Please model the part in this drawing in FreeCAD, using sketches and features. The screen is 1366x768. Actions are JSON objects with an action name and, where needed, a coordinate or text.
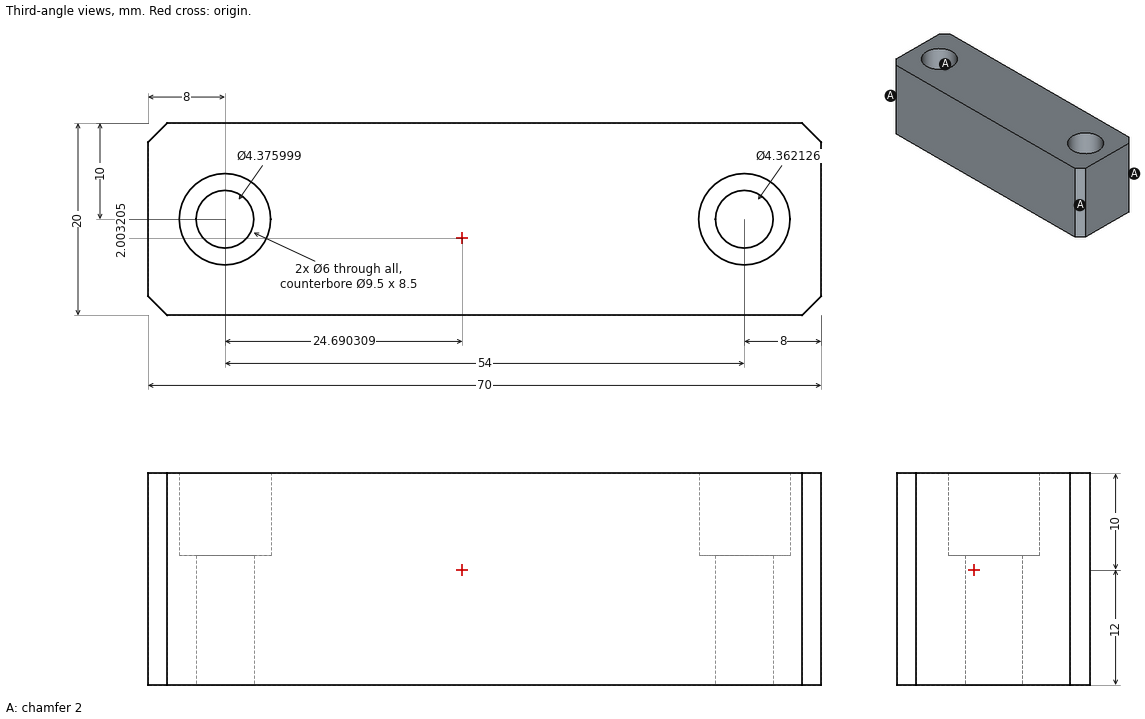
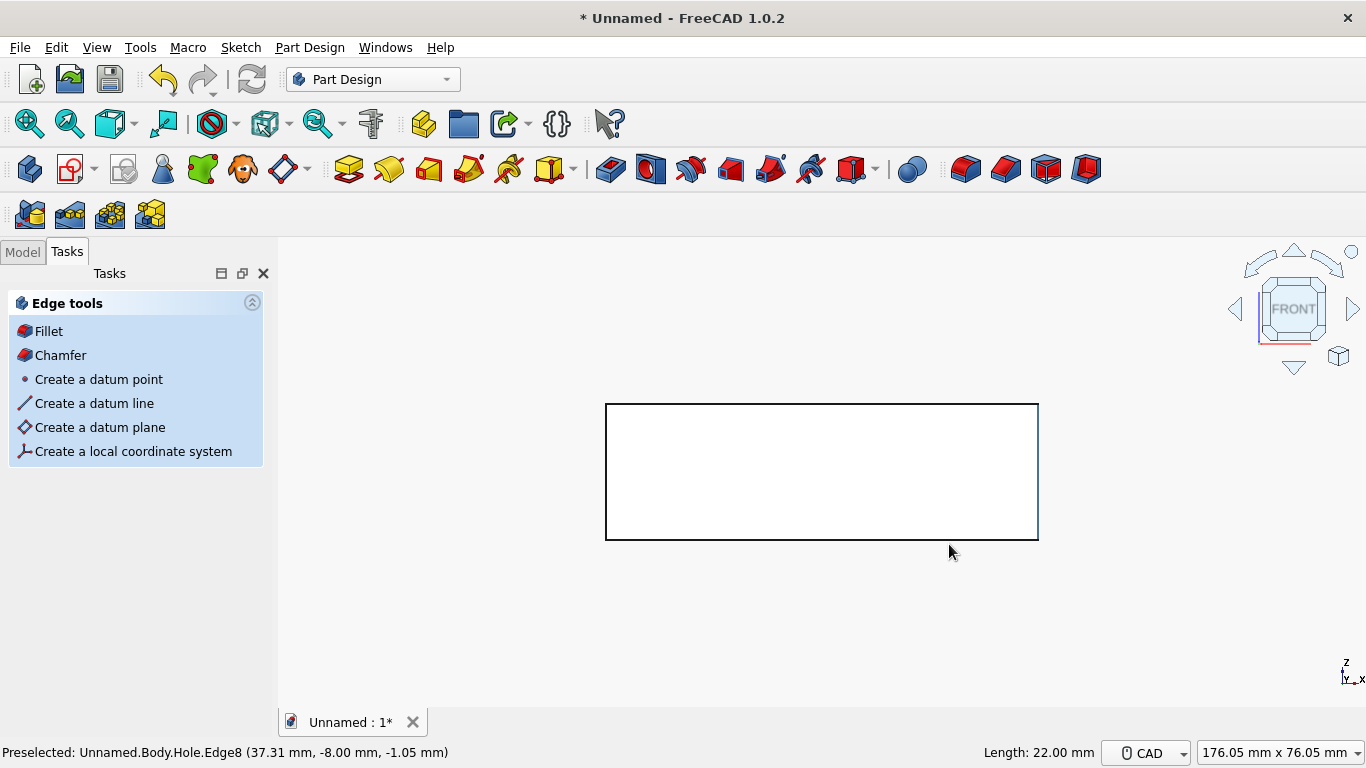
{"action": "left_click", "coordinate": [30, 124]}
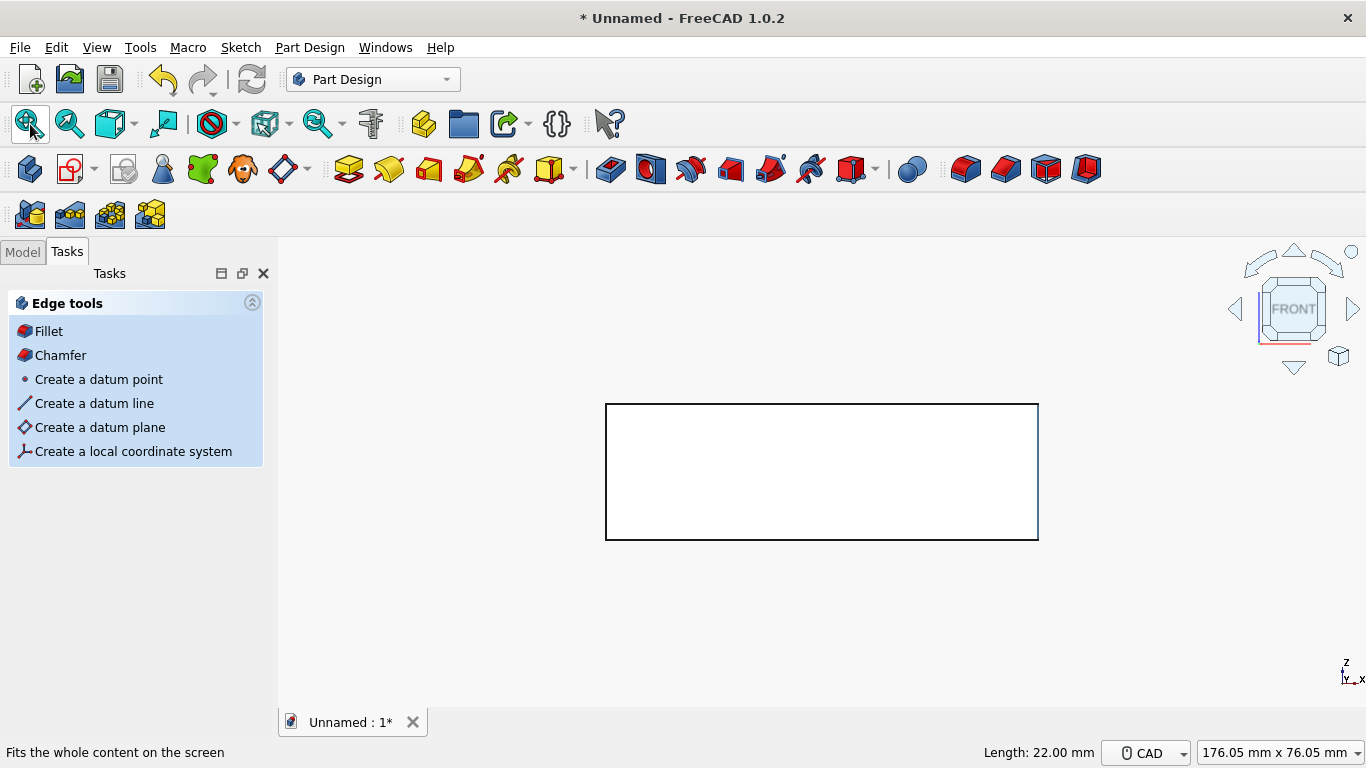
{"action": "left_click", "coordinate": [606, 471], "text": "ctrl"}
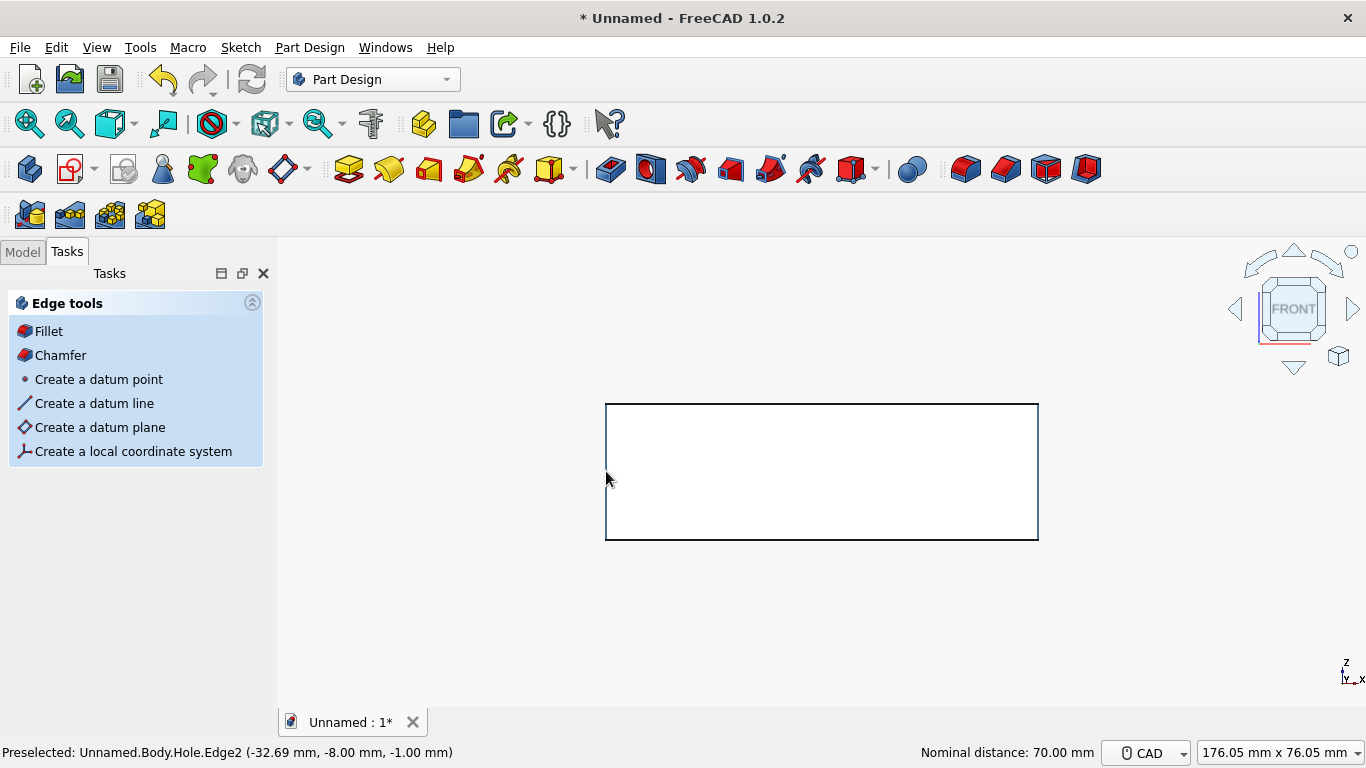
{"action": "key", "text": "3"}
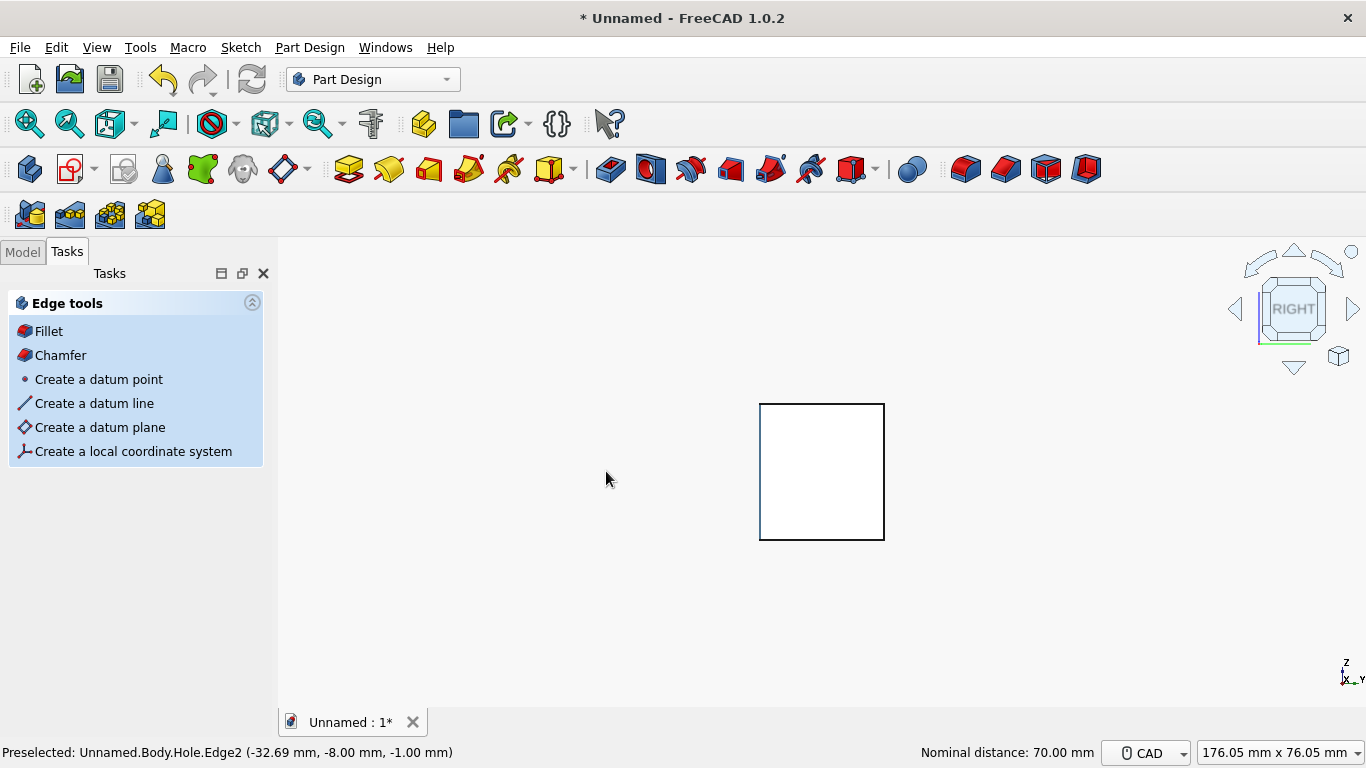
{"action": "key", "text": "v f"}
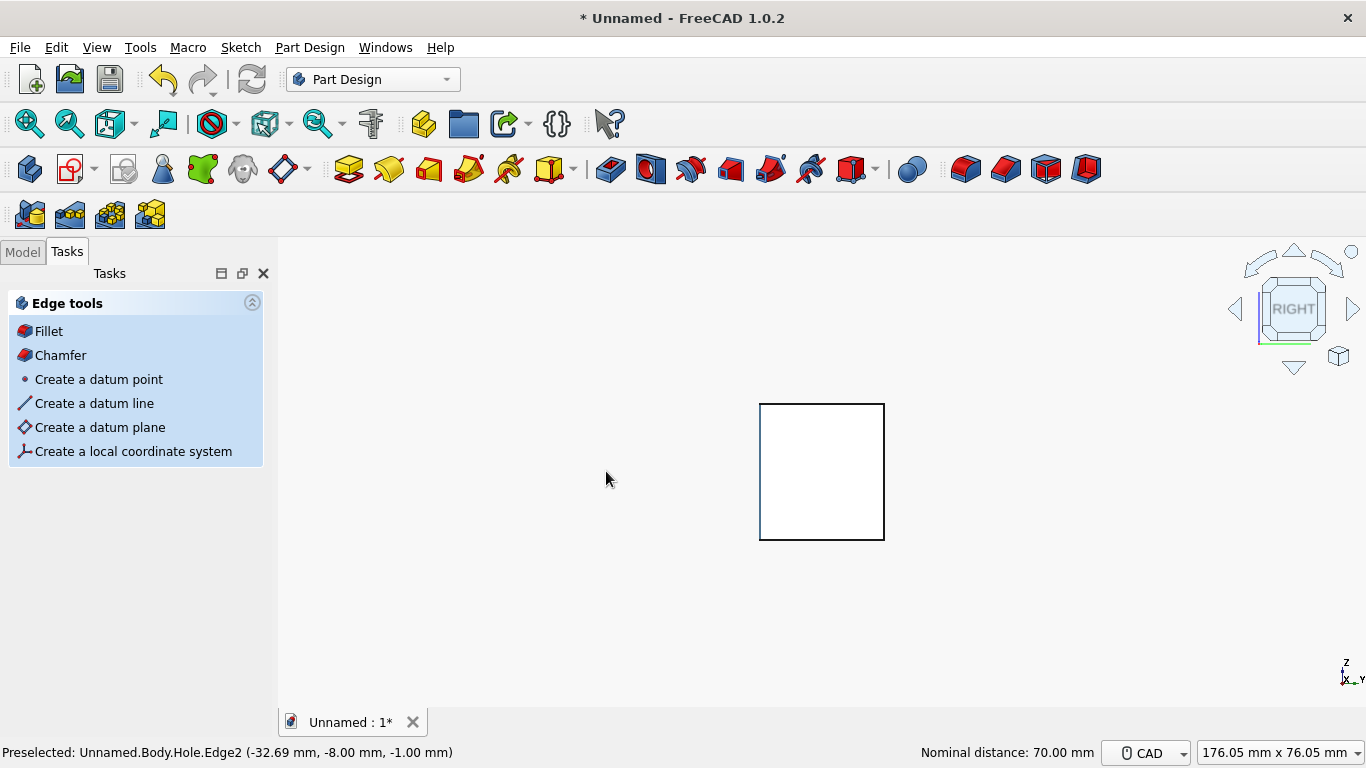
{"action": "left_click", "coordinate": [884, 471], "text": "ctrl"}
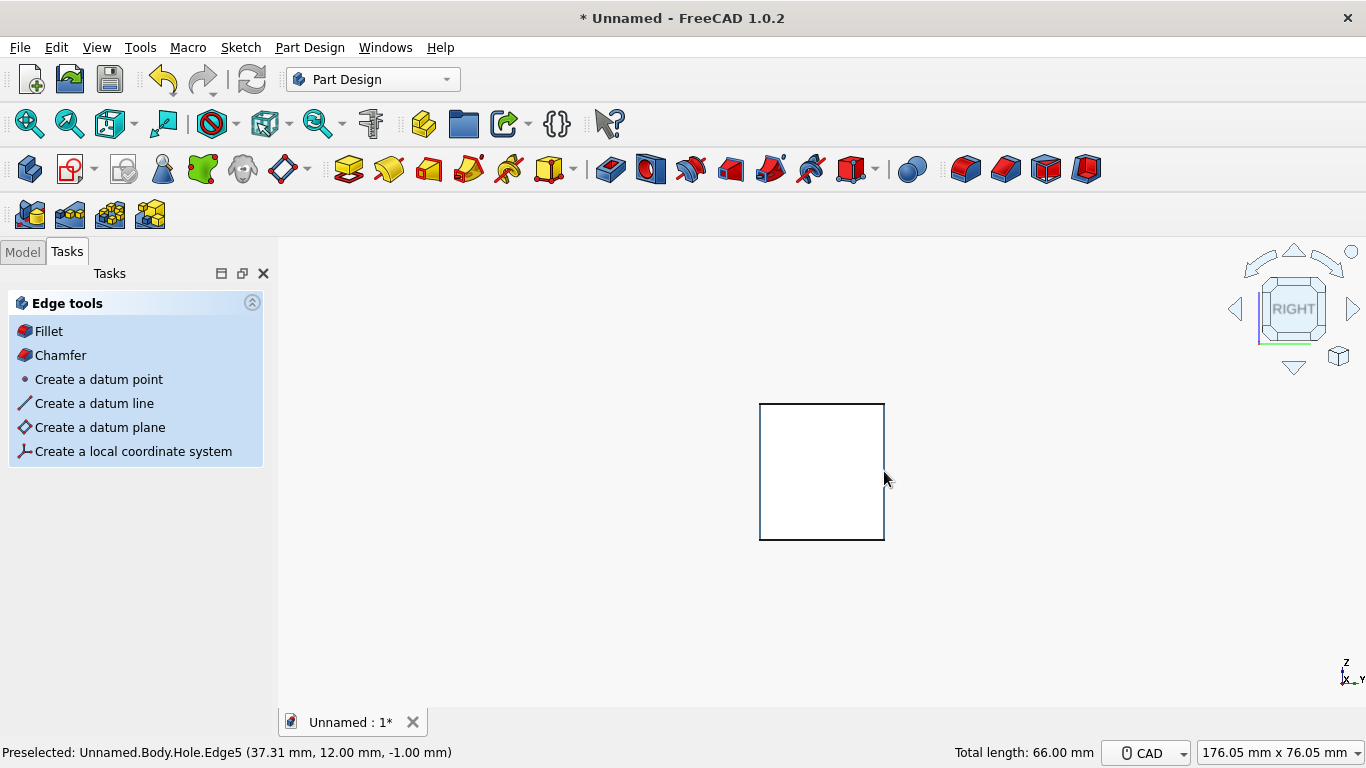
{"action": "key", "text": "5"}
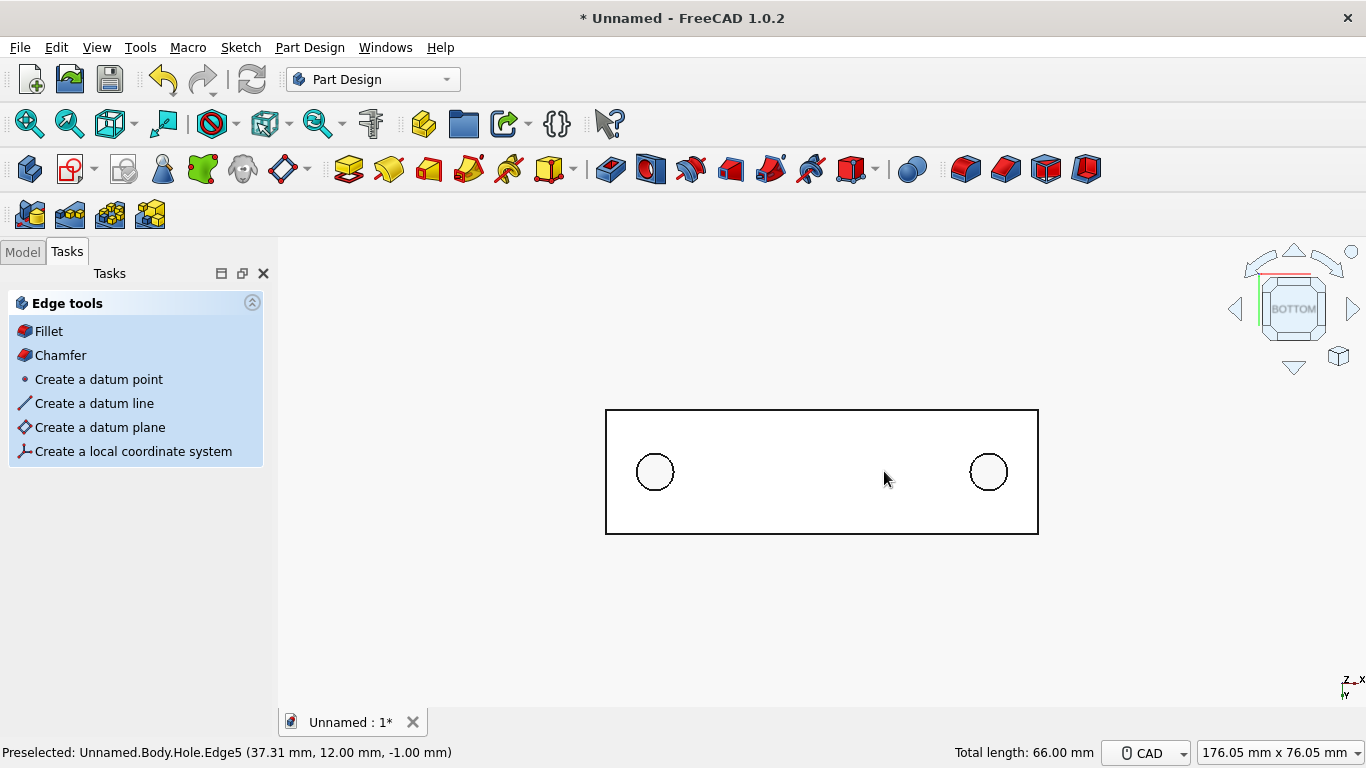
{"action": "key", "text": "v f"}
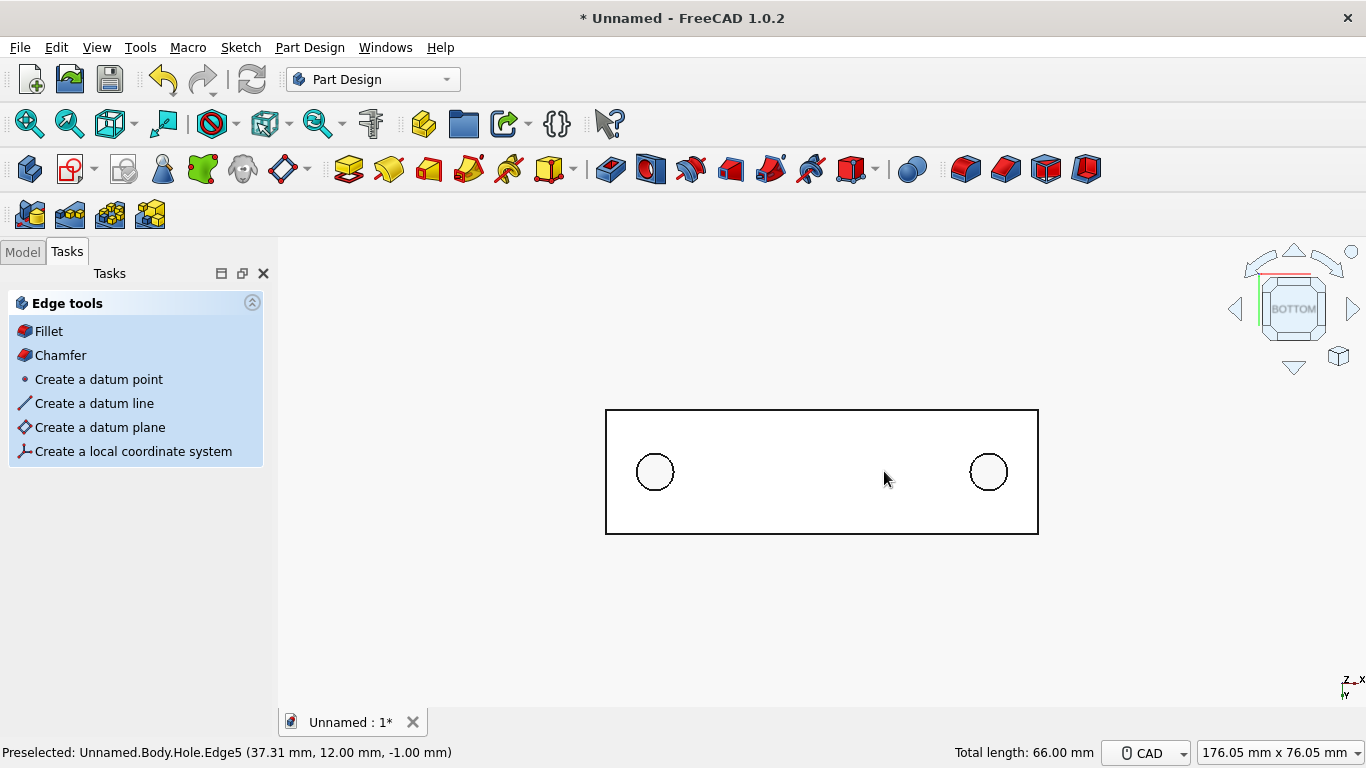
{"action": "key", "text": "4"}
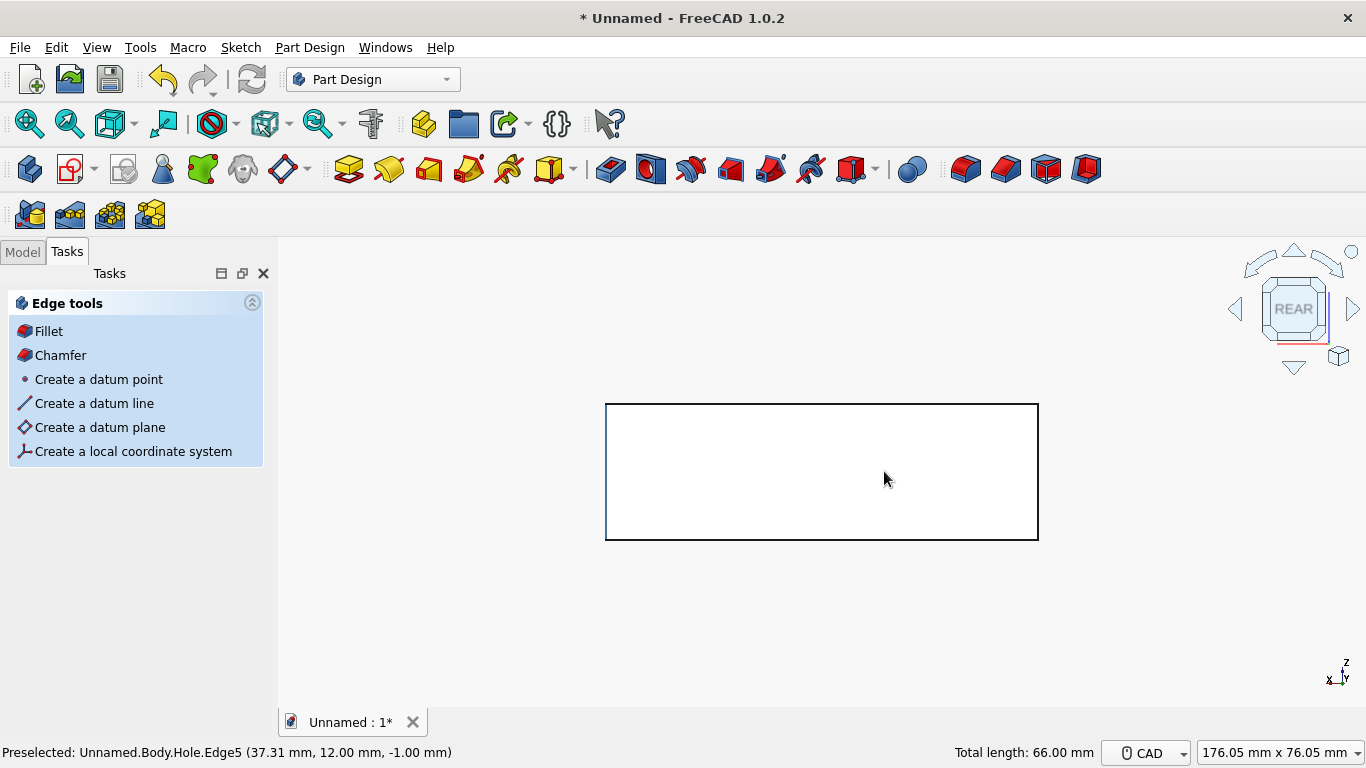
{"action": "key", "text": "v f"}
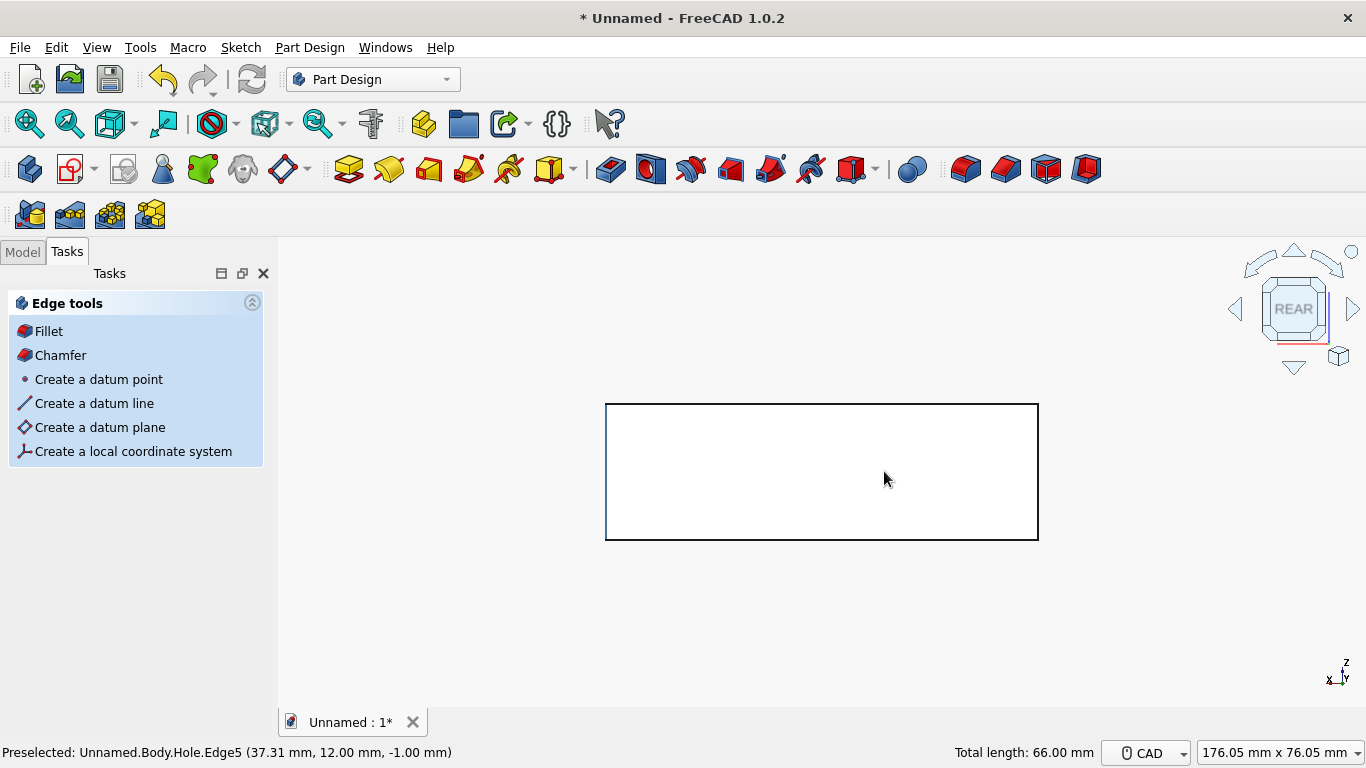
{"action": "left_click", "coordinate": [1038, 471], "text": "ctrl"}